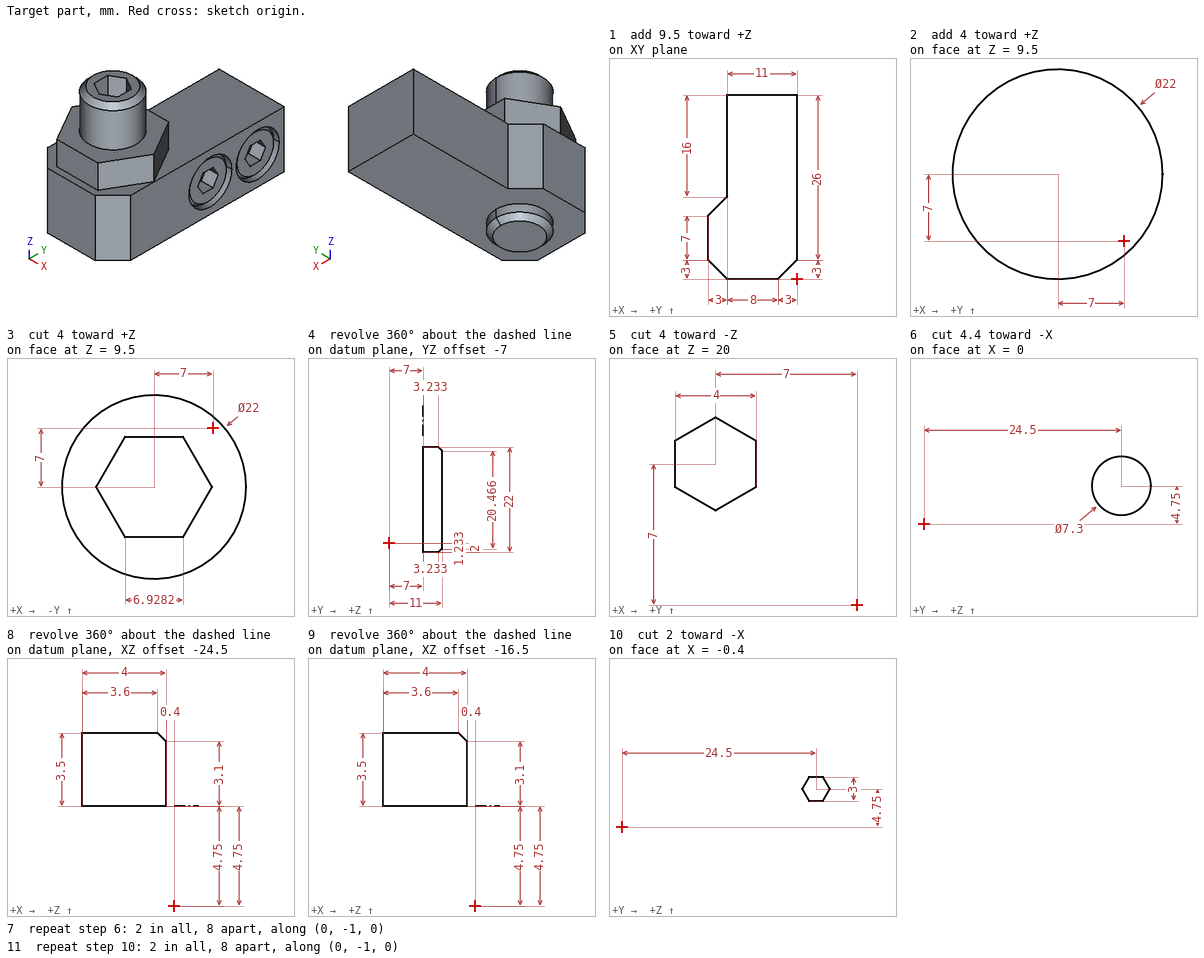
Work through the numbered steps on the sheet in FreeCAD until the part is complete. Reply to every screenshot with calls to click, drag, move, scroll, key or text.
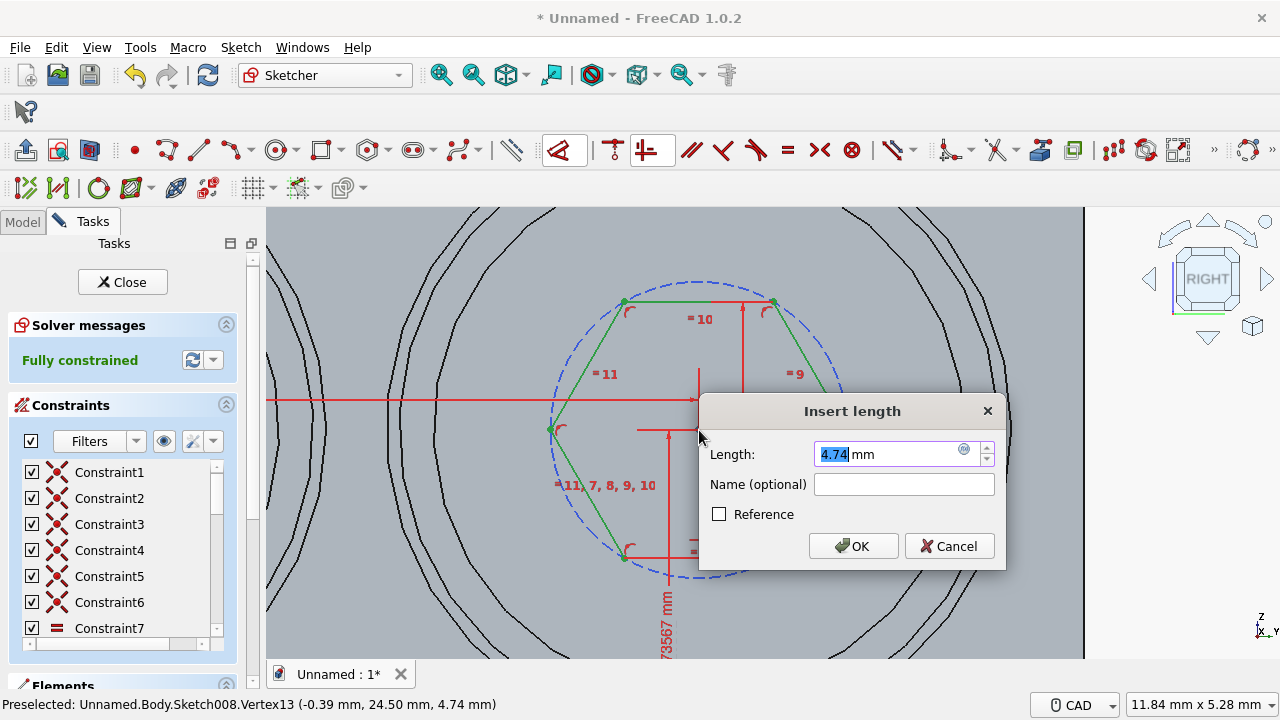
text(4.75)
key(Return)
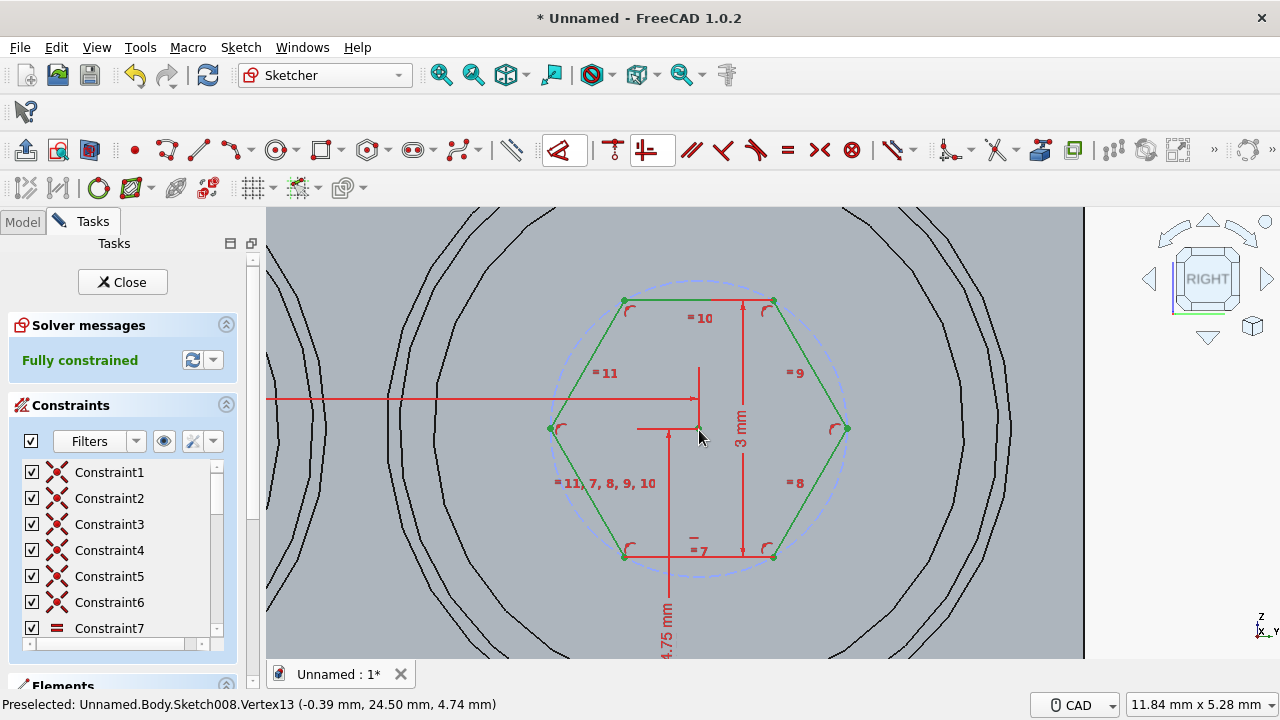
click(123, 282)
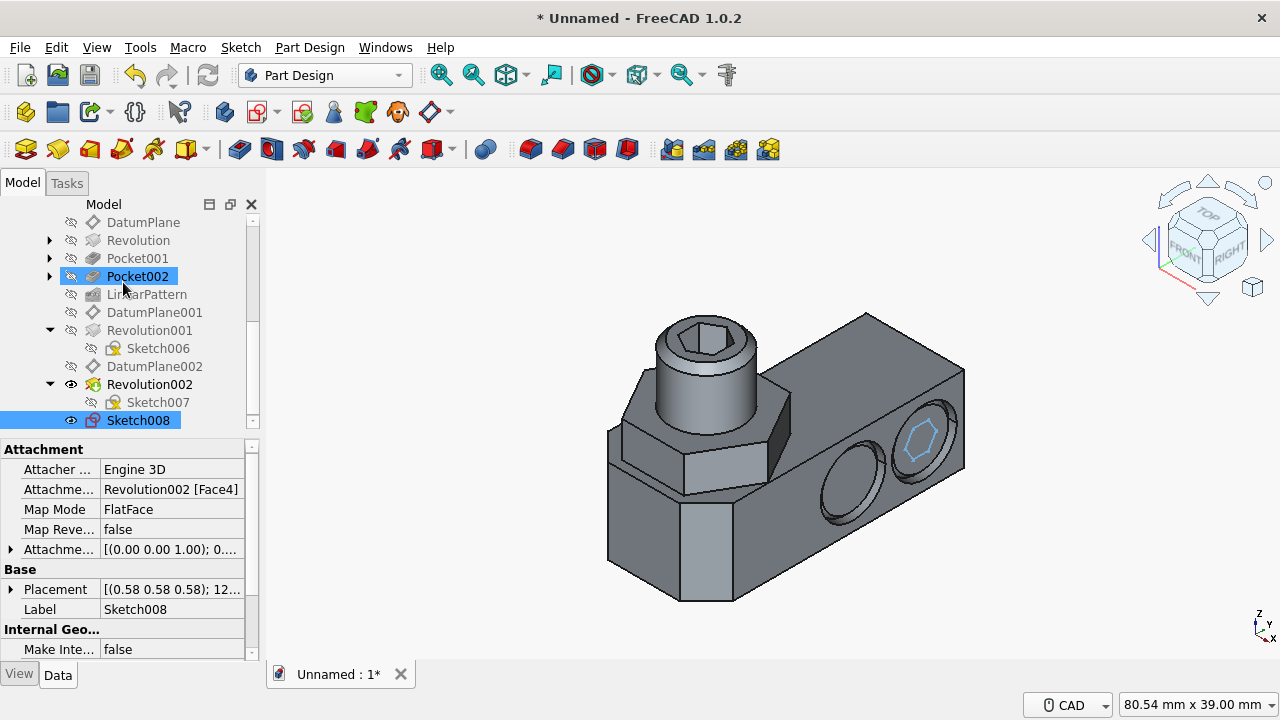
click(240, 150)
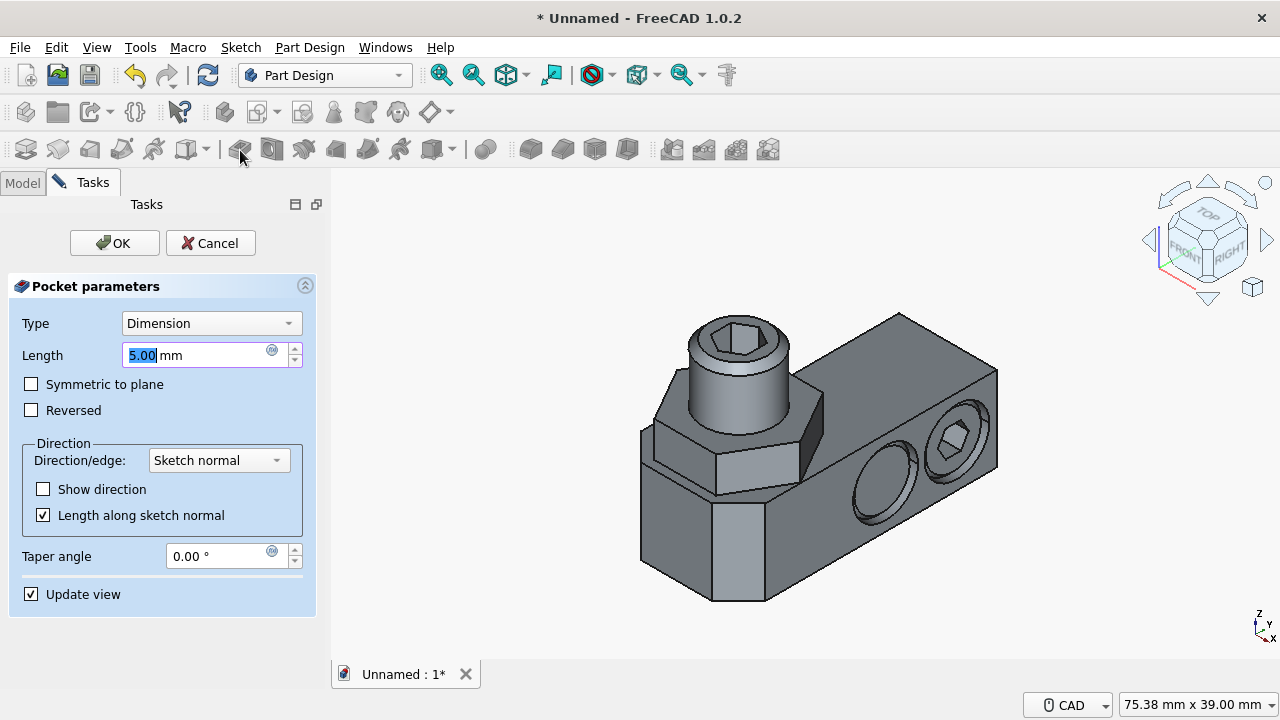
text(2)
key(Tab)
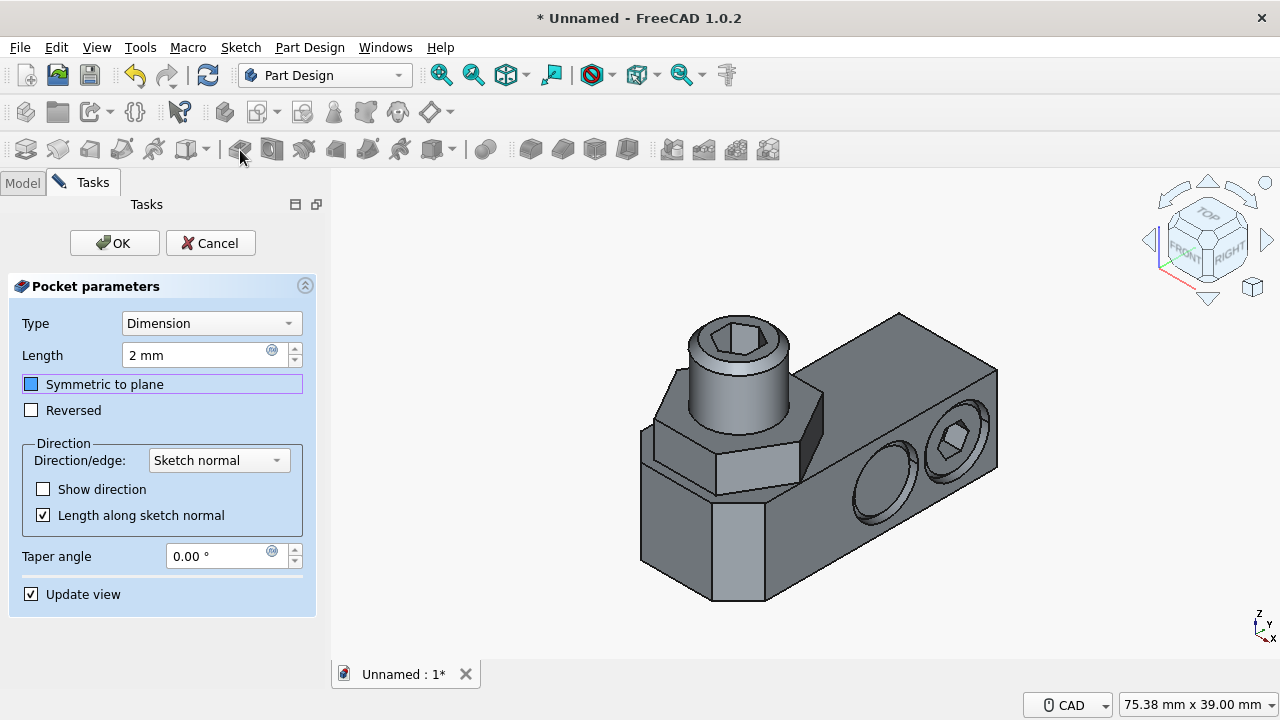
click(115, 243)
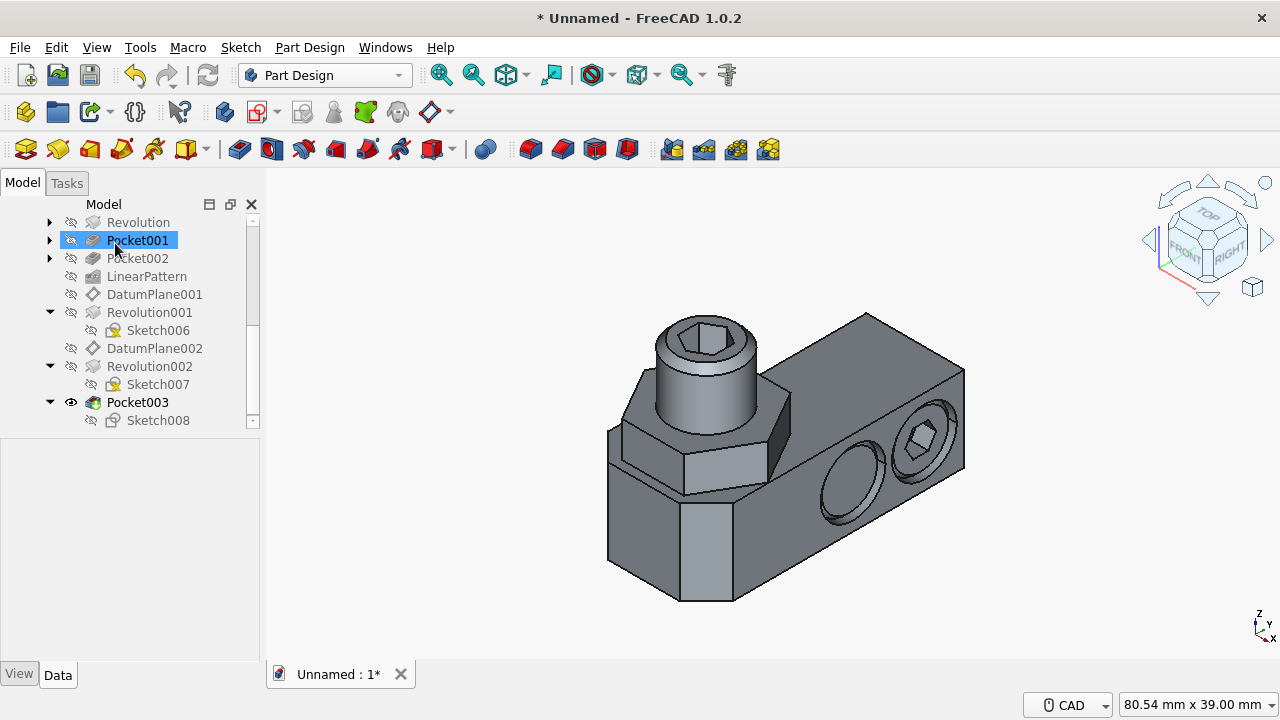
click(116, 402)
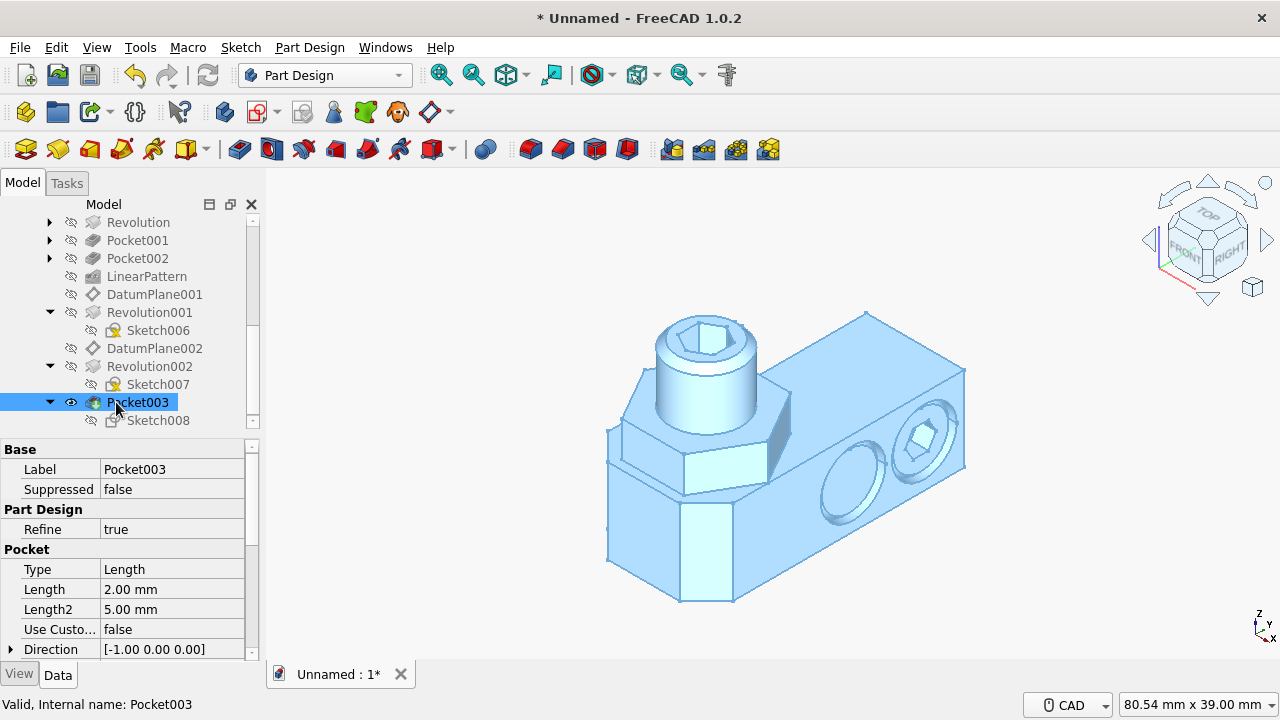
click(704, 150)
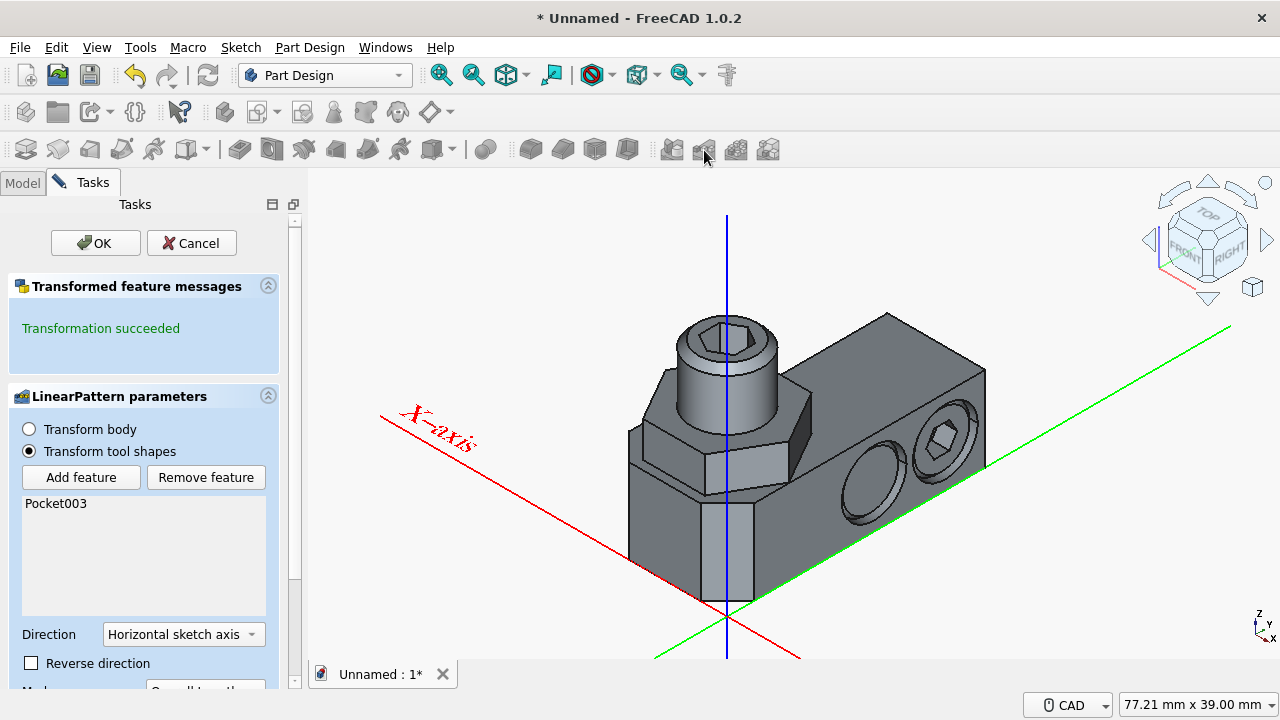
click(184, 634)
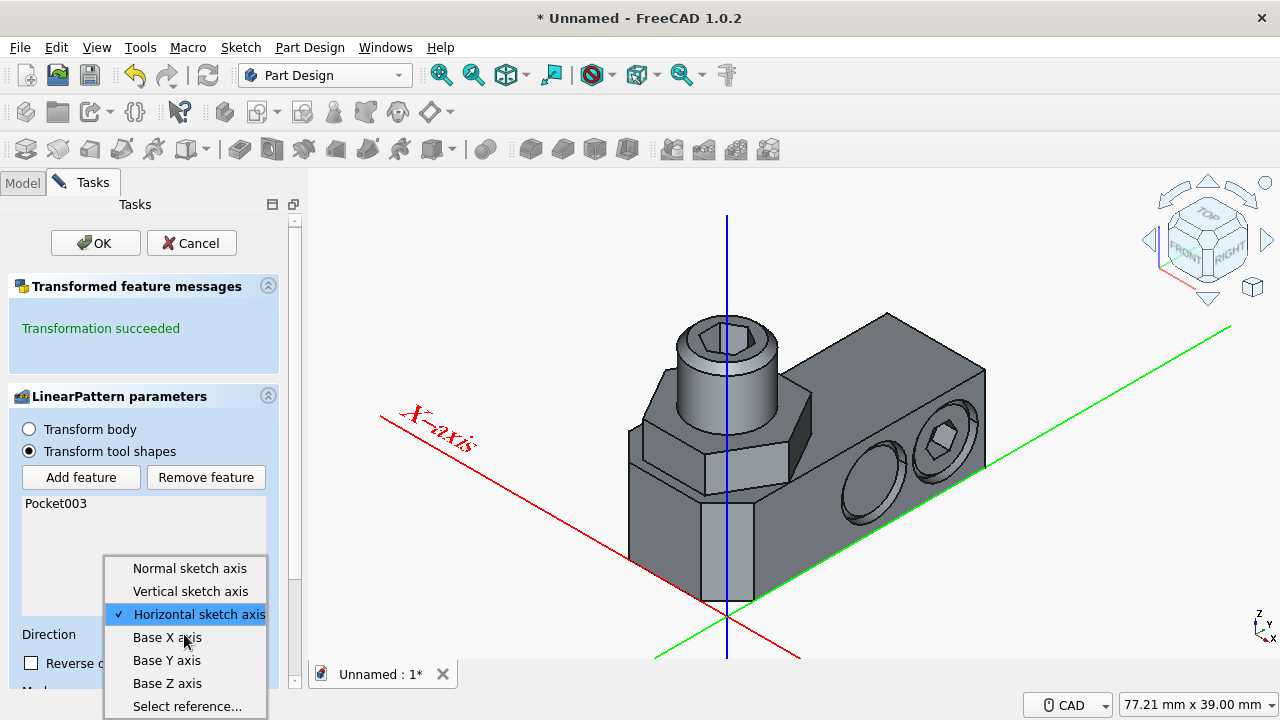
click(184, 660)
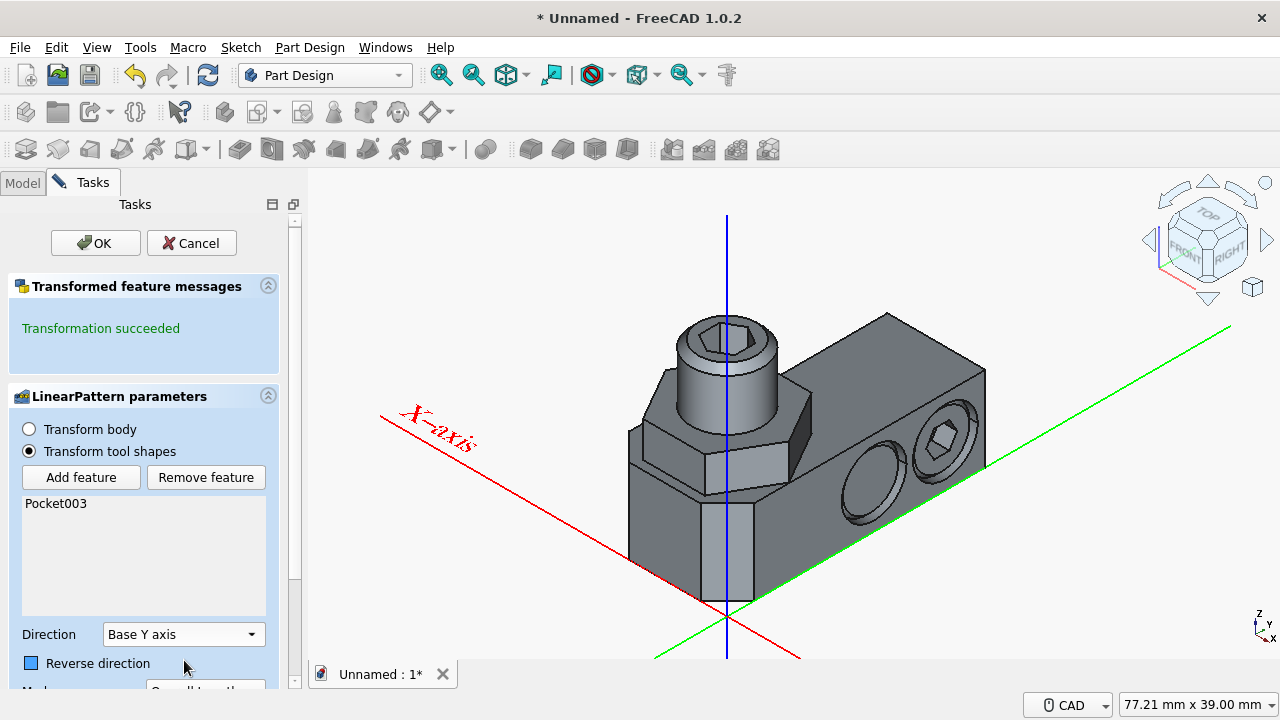
scroll(295, 451, down, 2)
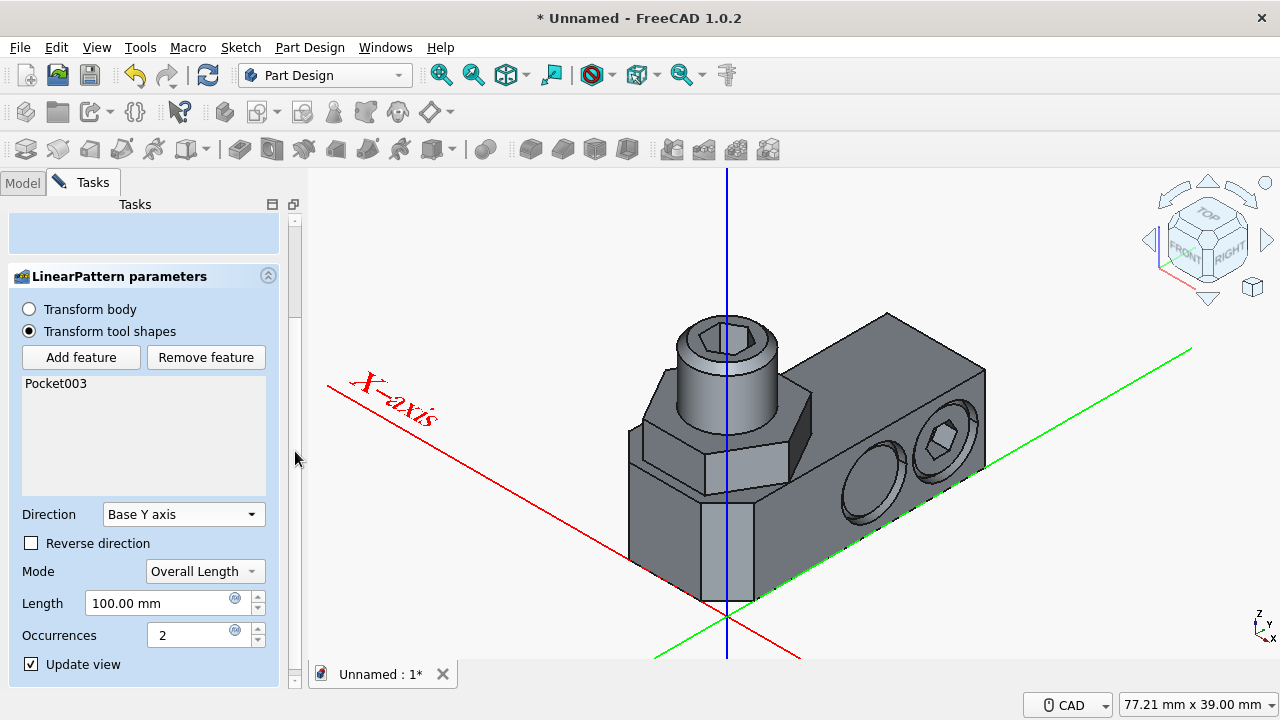
click(206, 572)